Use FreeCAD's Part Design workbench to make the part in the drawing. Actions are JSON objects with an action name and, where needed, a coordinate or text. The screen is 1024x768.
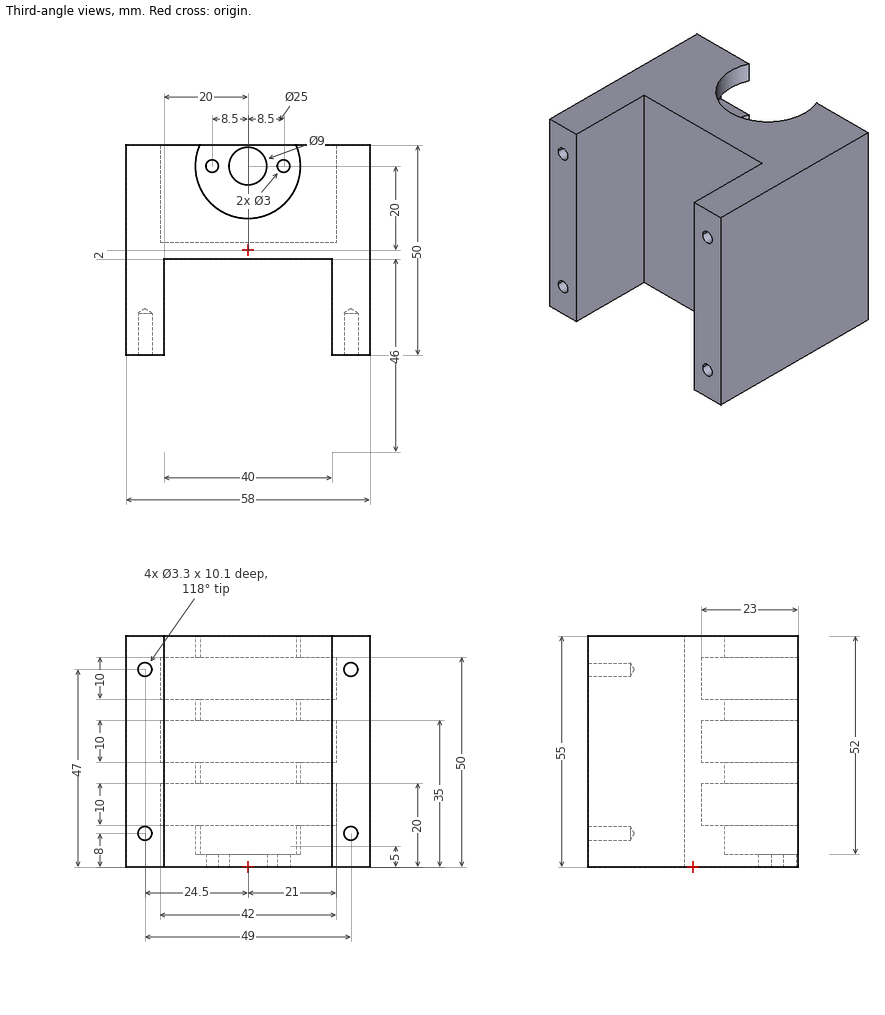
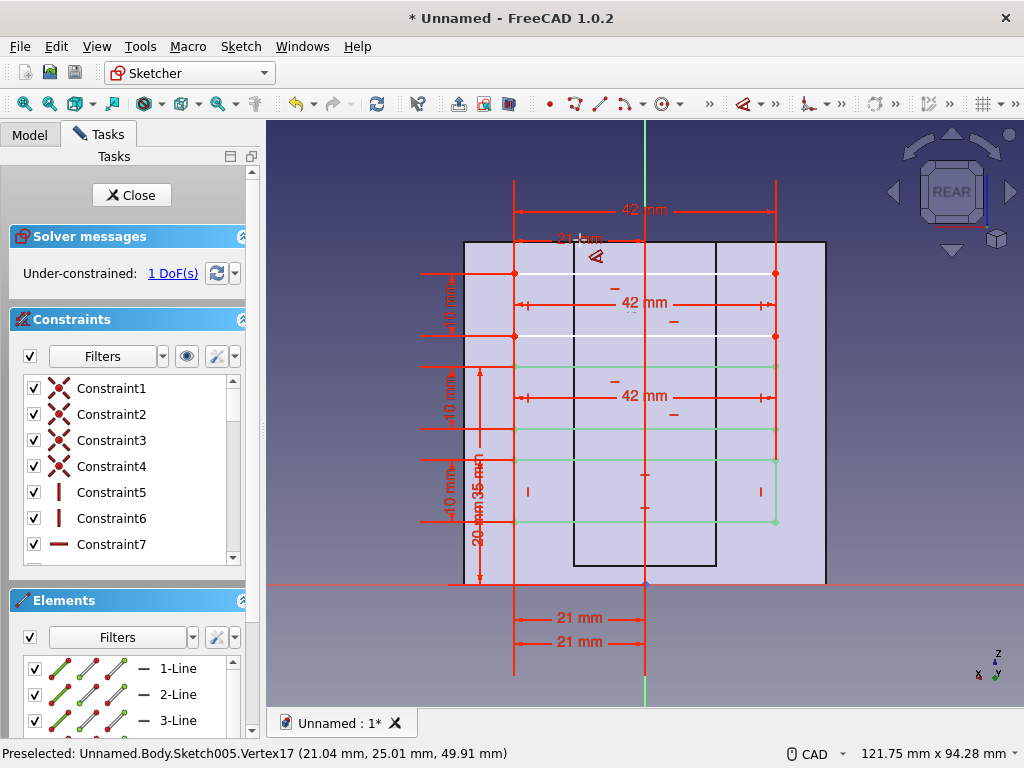
{"action": "left_click", "coordinate": [514, 274]}
{"action": "left_click", "coordinate": [480, 429]}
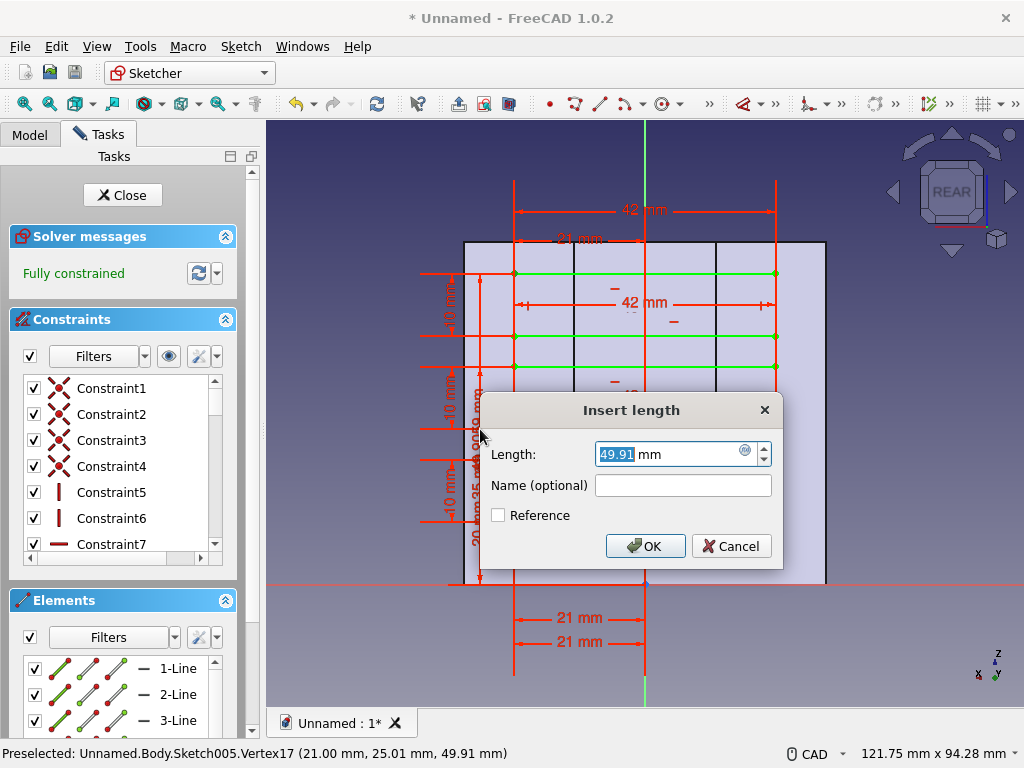
{"action": "type", "text": "50"}
{"action": "key", "text": "Return"}
{"action": "key", "text": "Escape"}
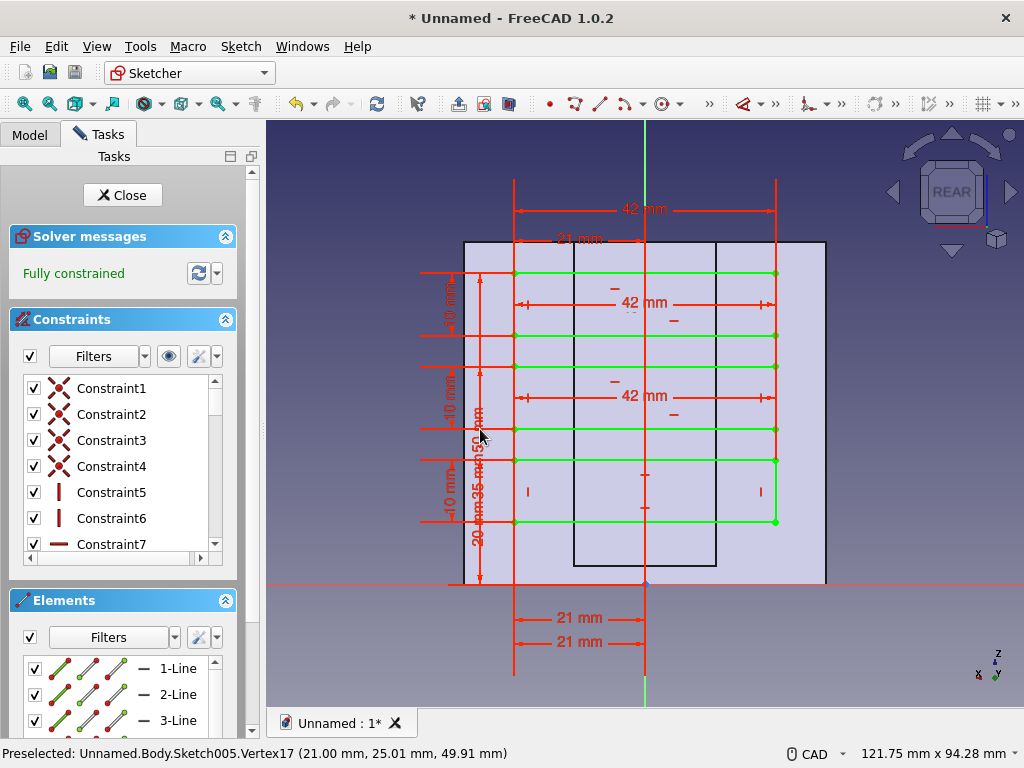
{"action": "left_click", "coordinate": [123, 195]}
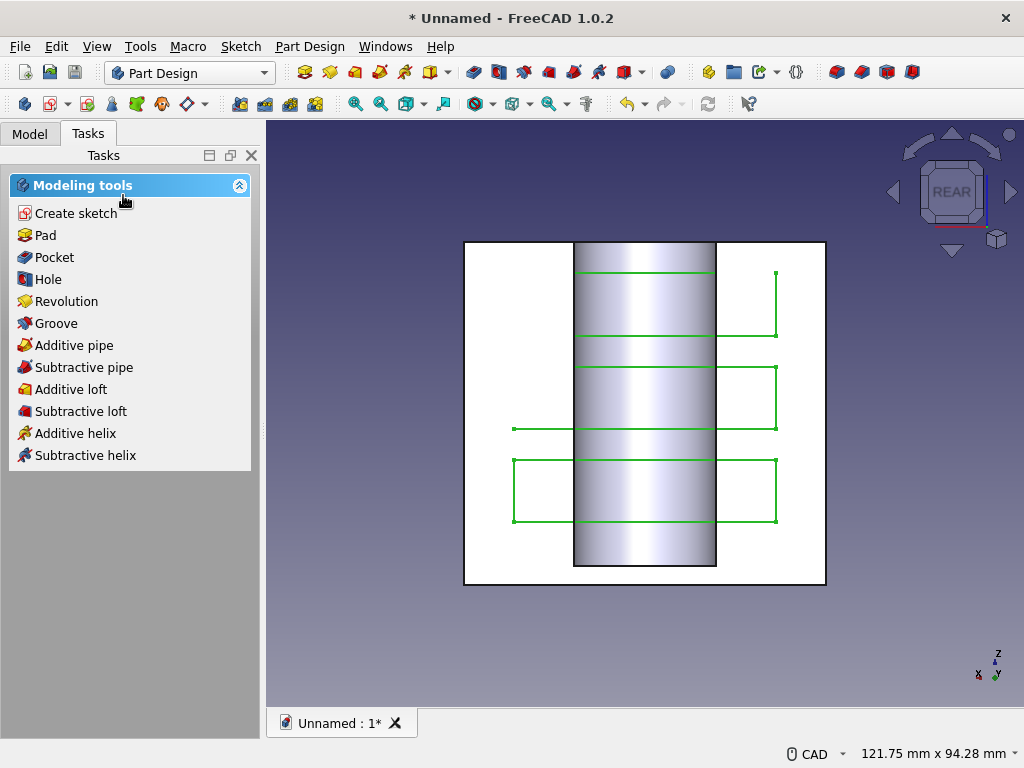
{"action": "left_click", "coordinate": [474, 72]}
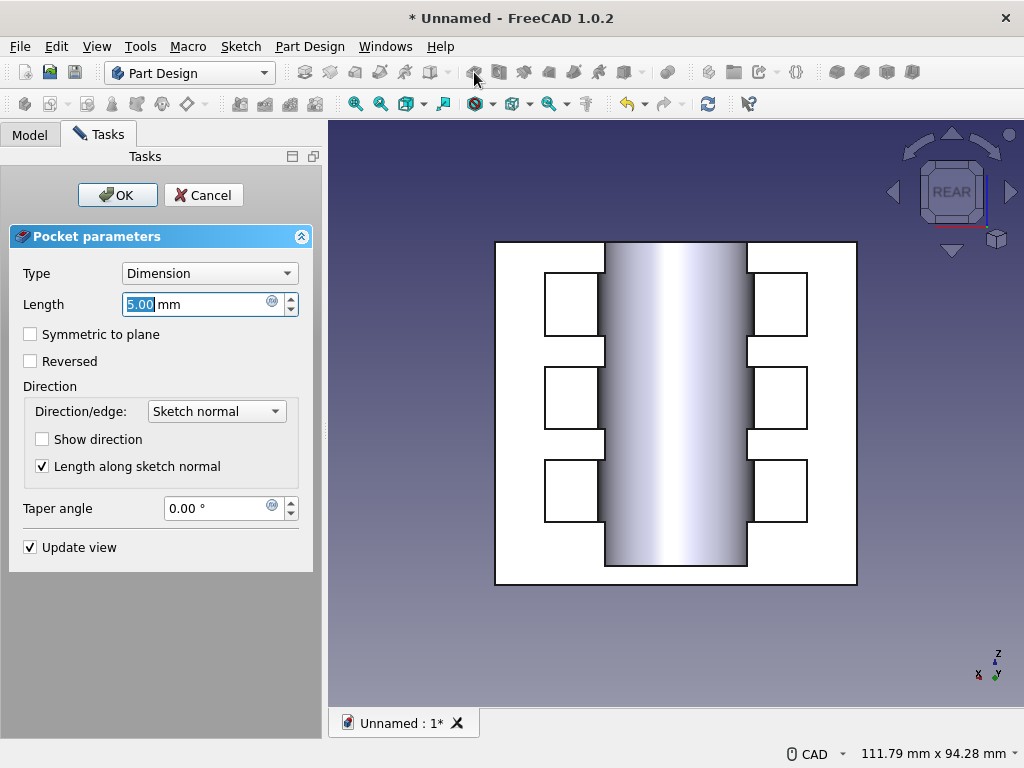
{"action": "type", "text": "23"}
{"action": "key", "text": "Tab"}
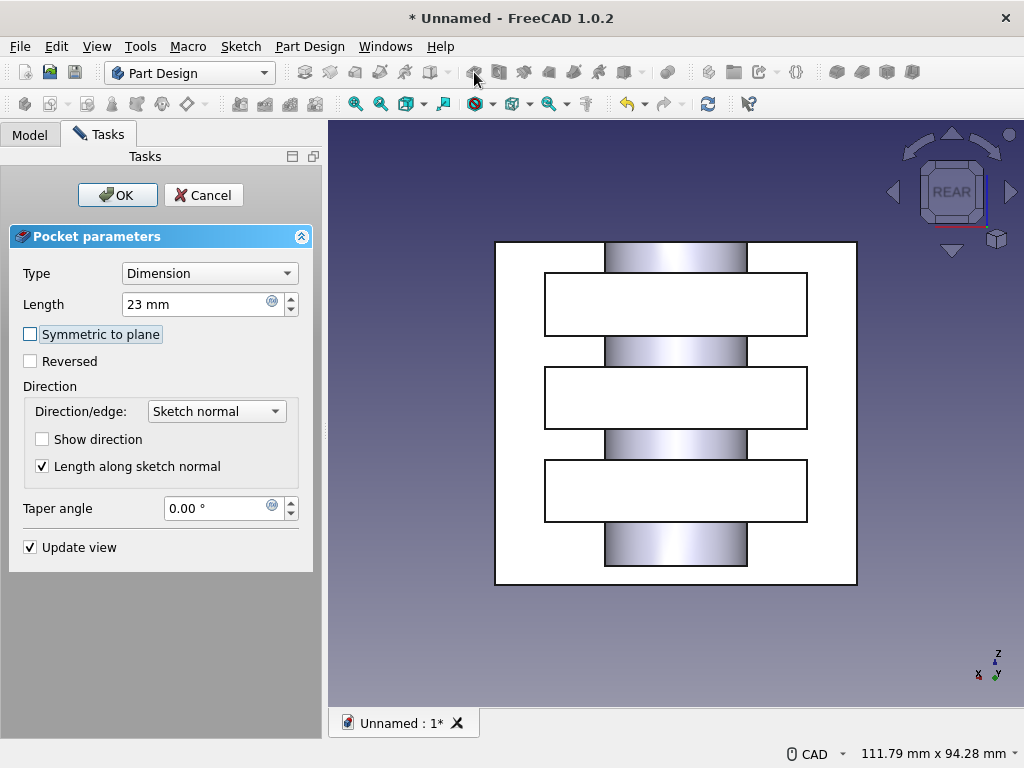
{"action": "left_click", "coordinate": [118, 195]}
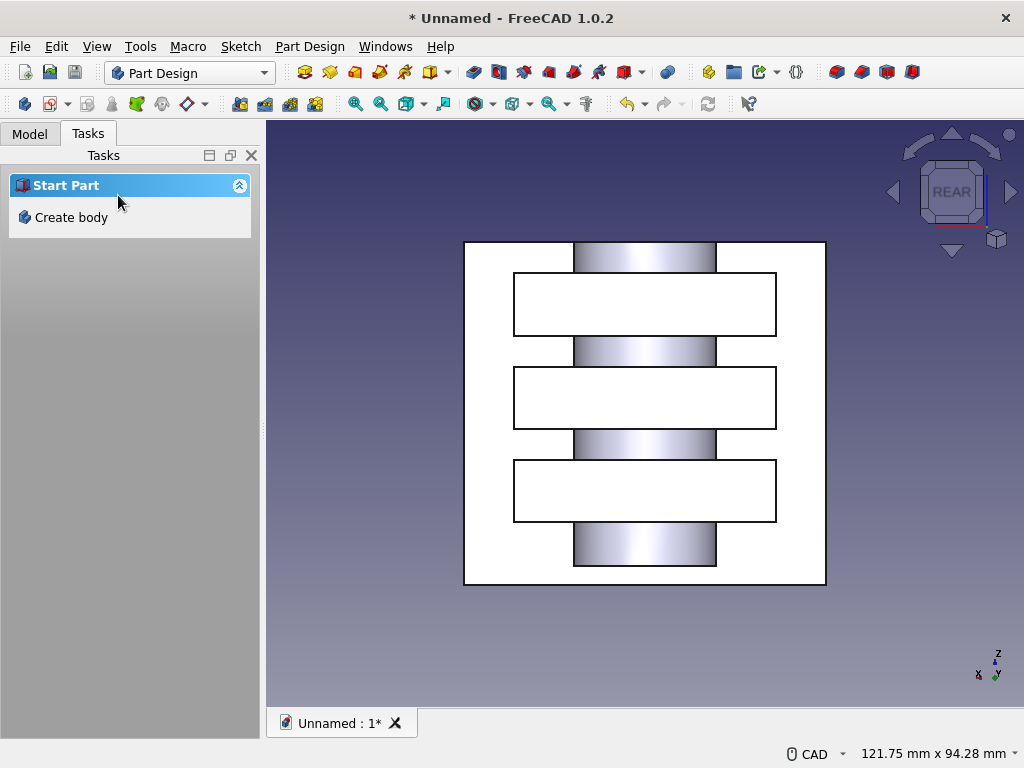
{"action": "key", "text": "0"}